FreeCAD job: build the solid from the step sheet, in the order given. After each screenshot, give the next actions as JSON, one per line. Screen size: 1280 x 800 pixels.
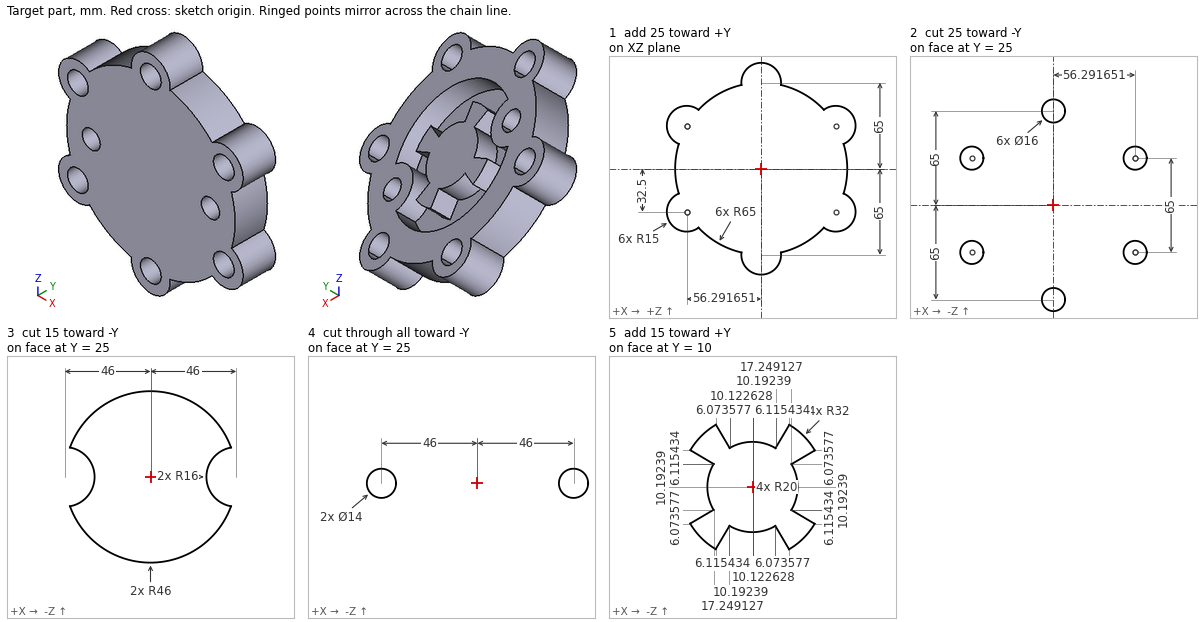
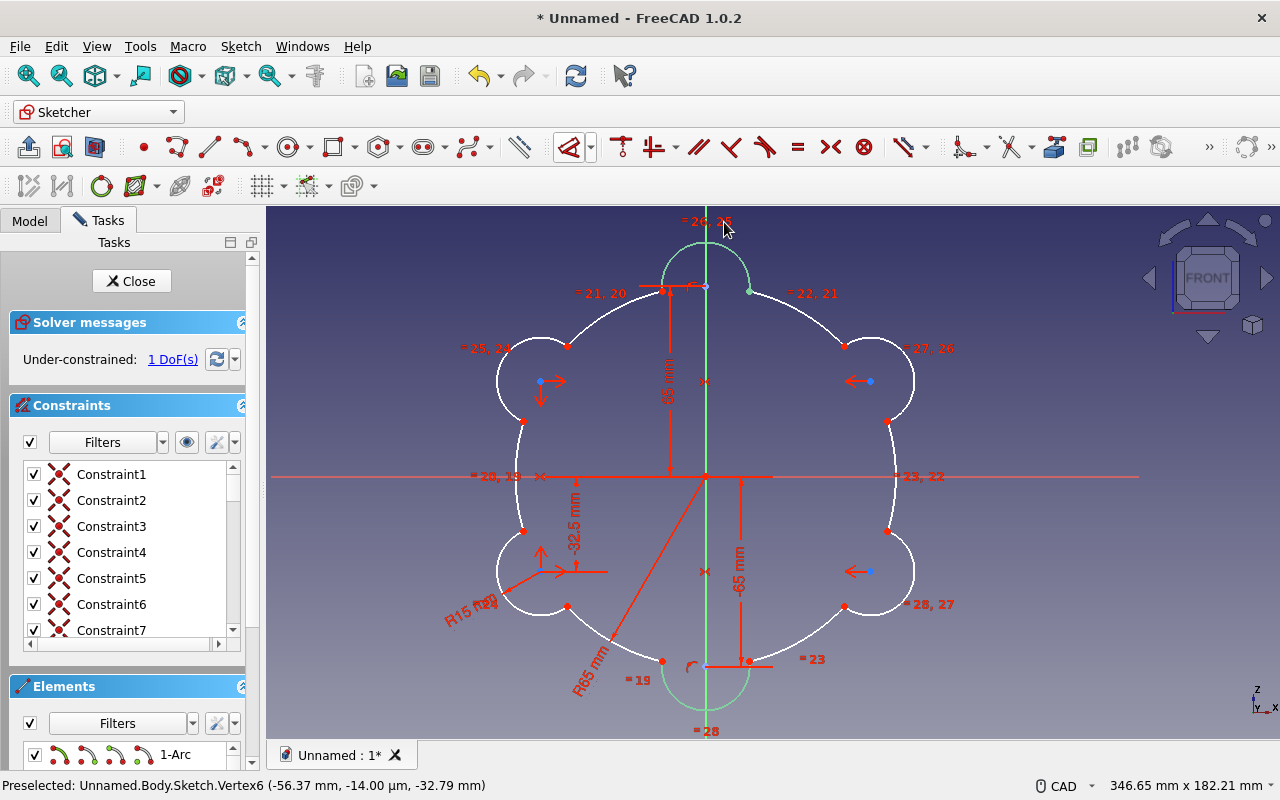
{"action": "left_click", "coordinate": [541, 572]}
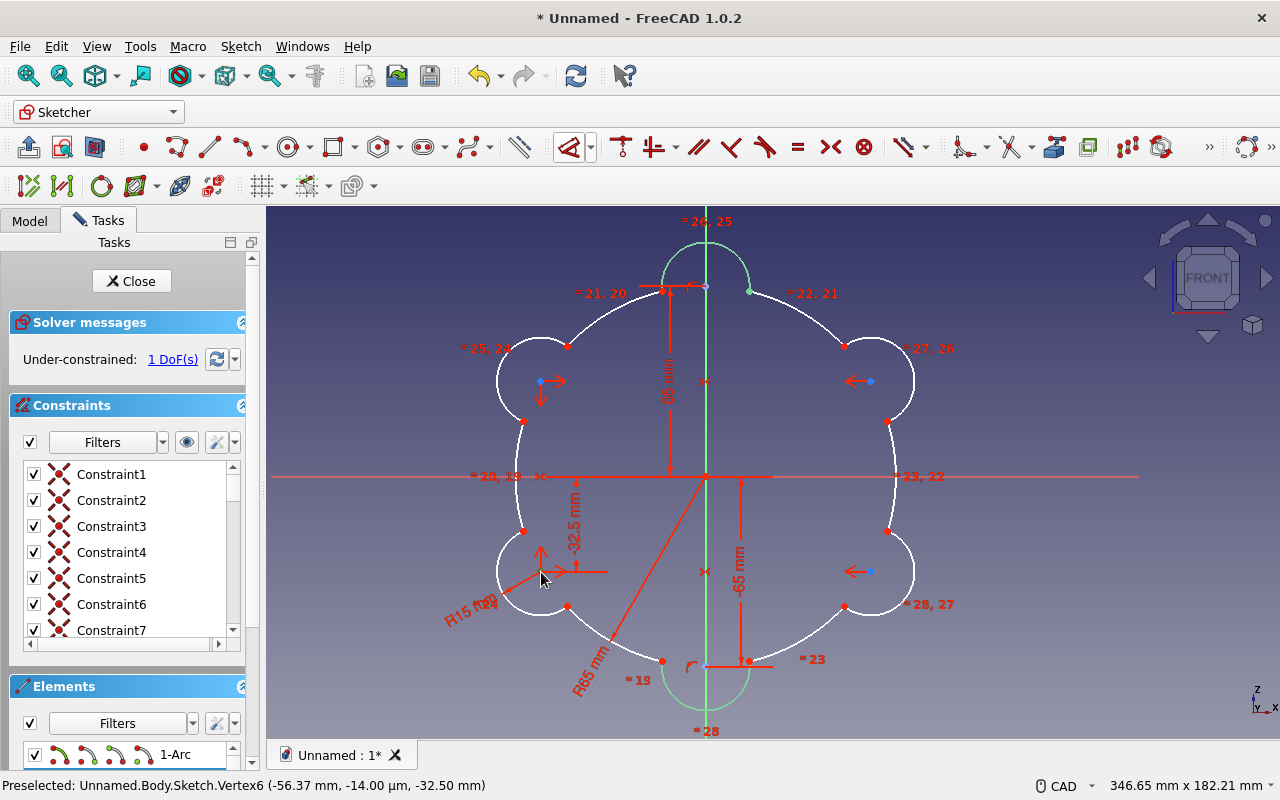
{"action": "left_click", "coordinate": [590, 148]}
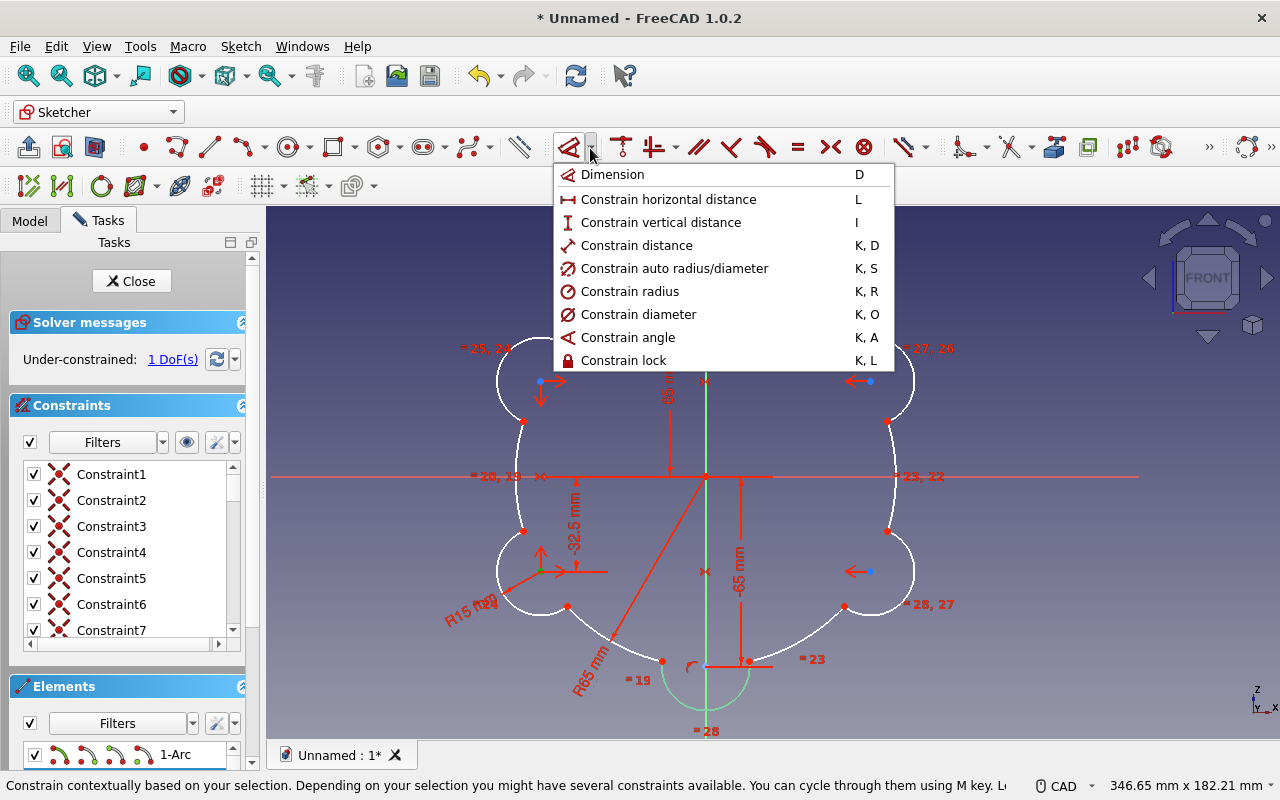
{"action": "left_click", "coordinate": [724, 200]}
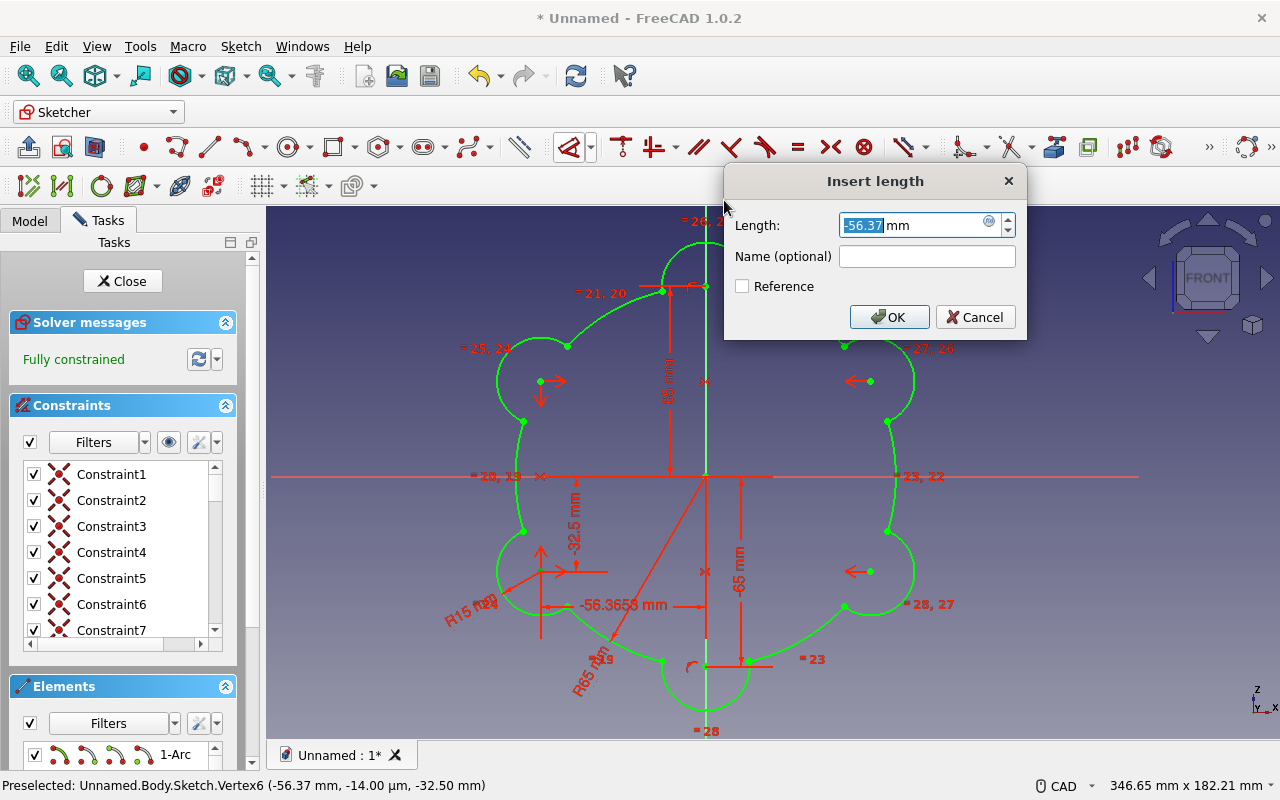
{"action": "type", "text": "-56.291651"}
{"action": "key", "text": "Return"}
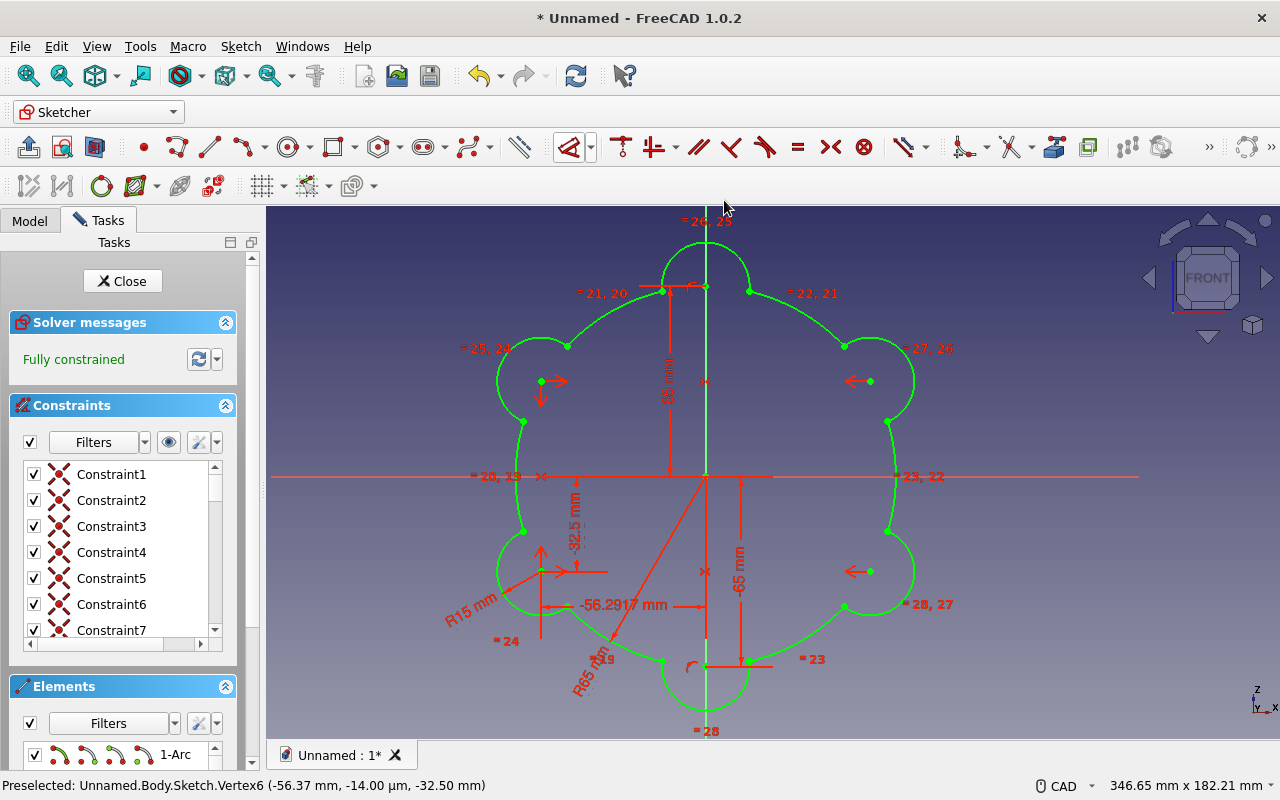
{"action": "left_click", "coordinate": [123, 281]}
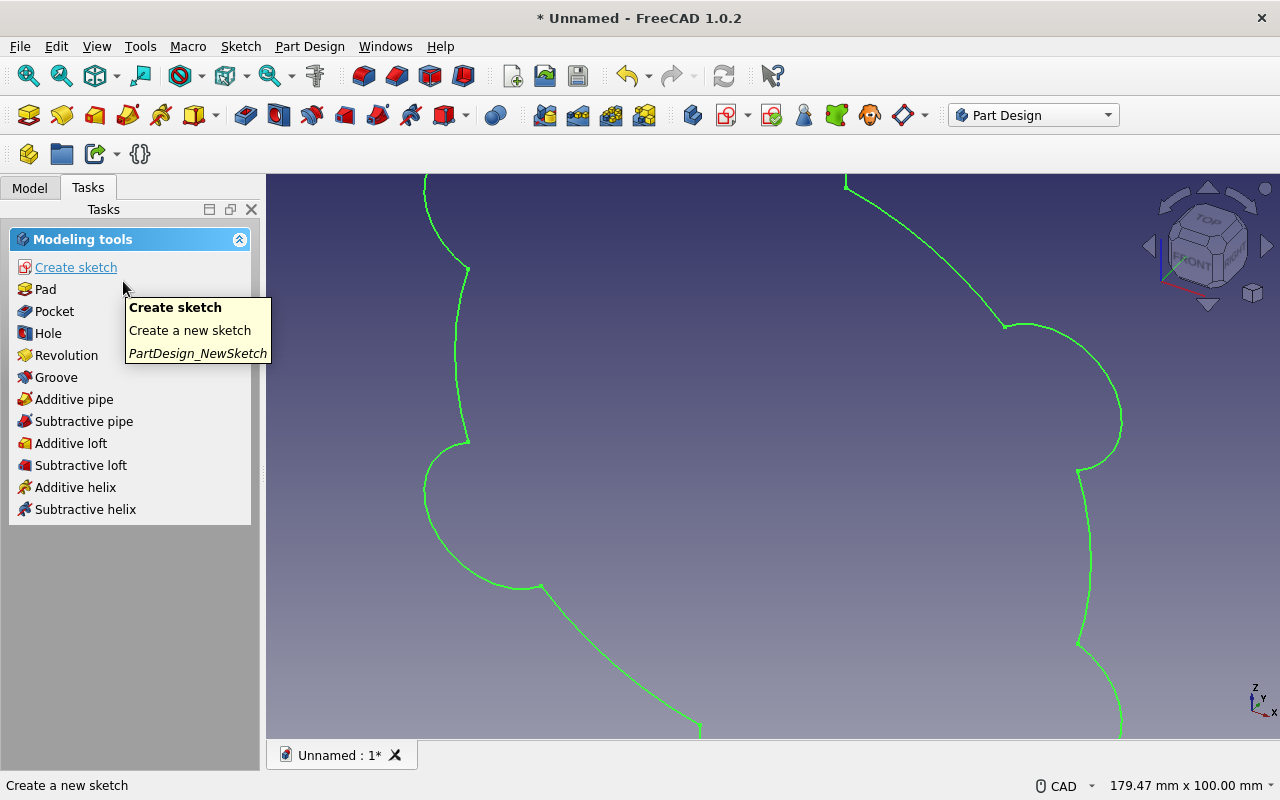
{"action": "left_click", "coordinate": [29, 116]}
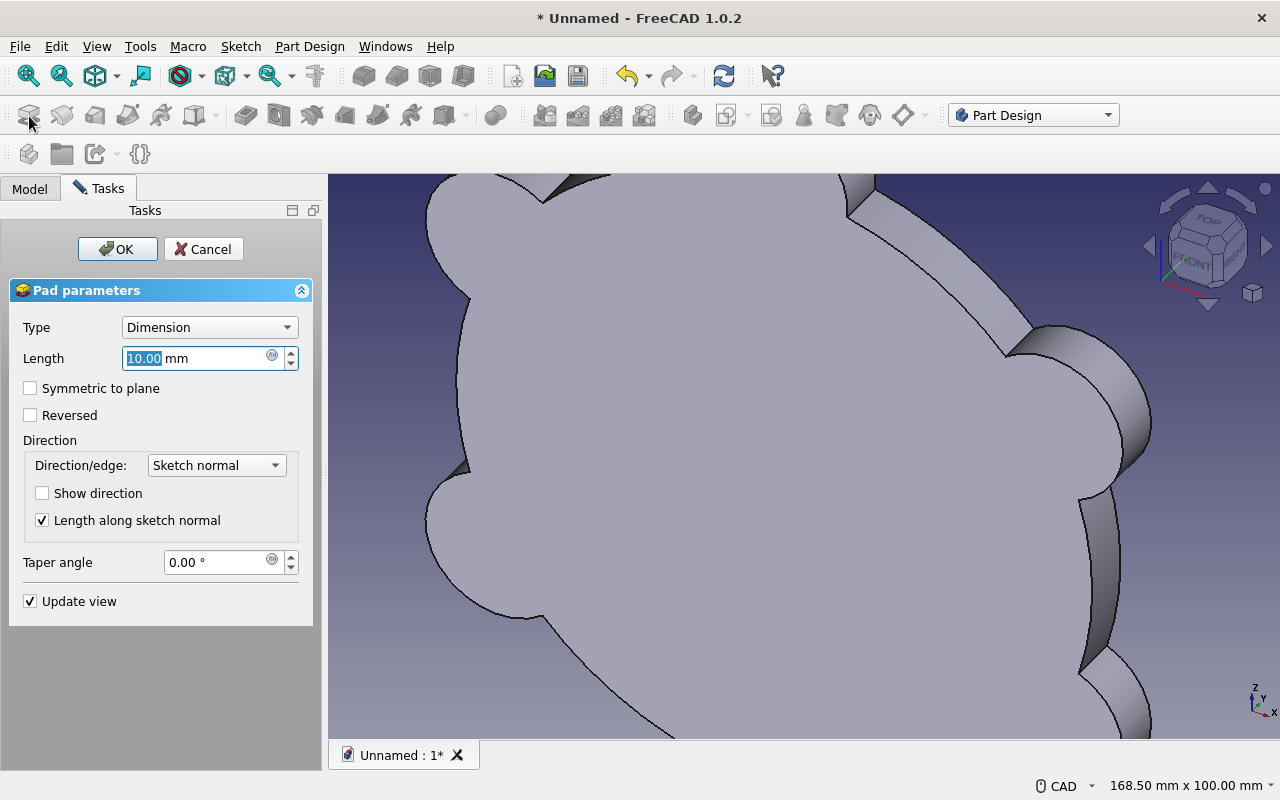
{"action": "type", "text": "25"}
{"action": "key", "text": "Tab"}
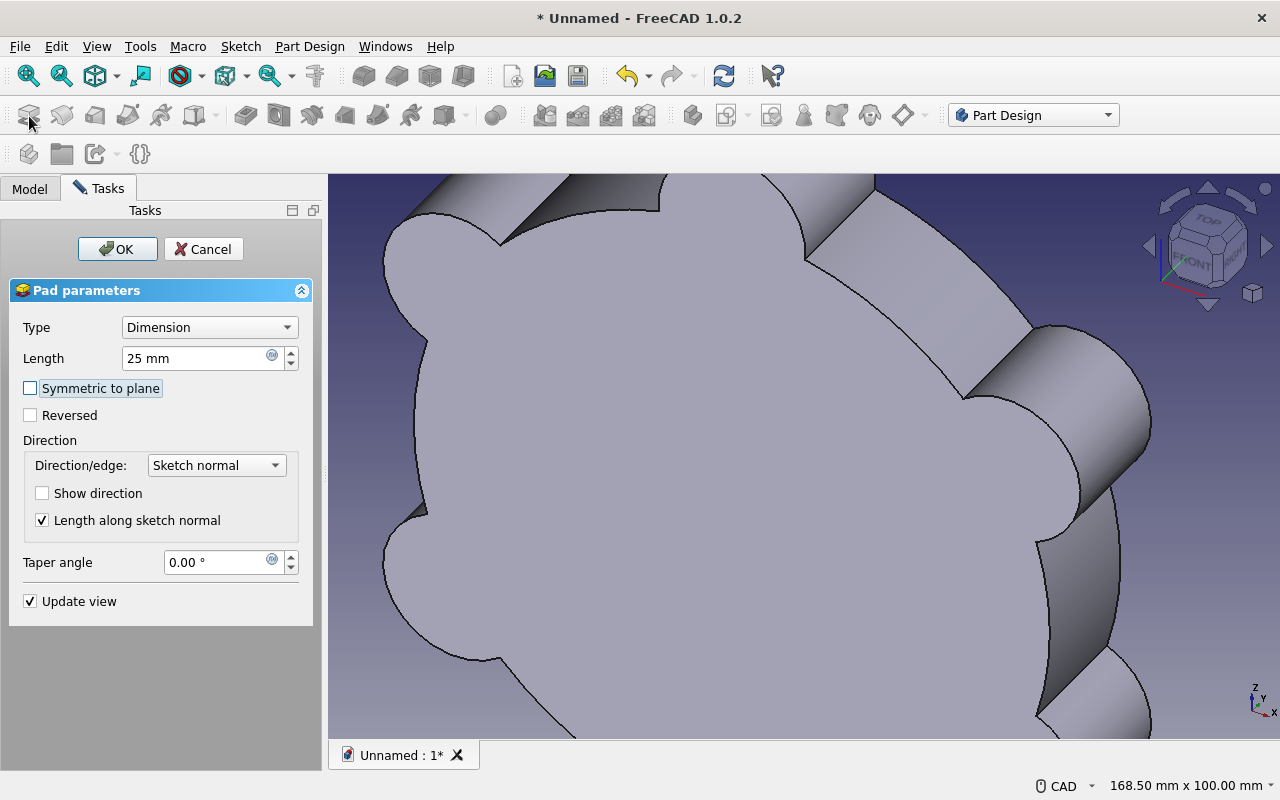
{"action": "left_click", "coordinate": [31, 415]}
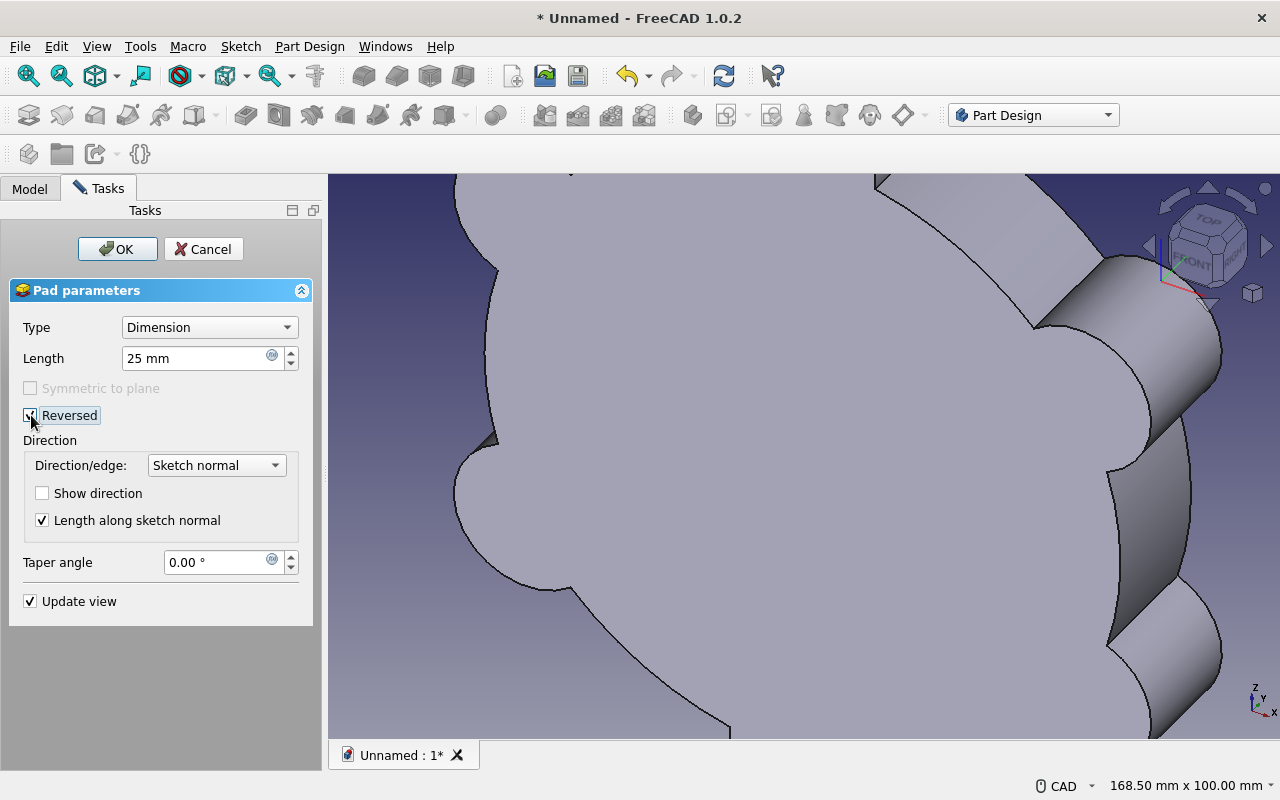
{"action": "left_click", "coordinate": [118, 249]}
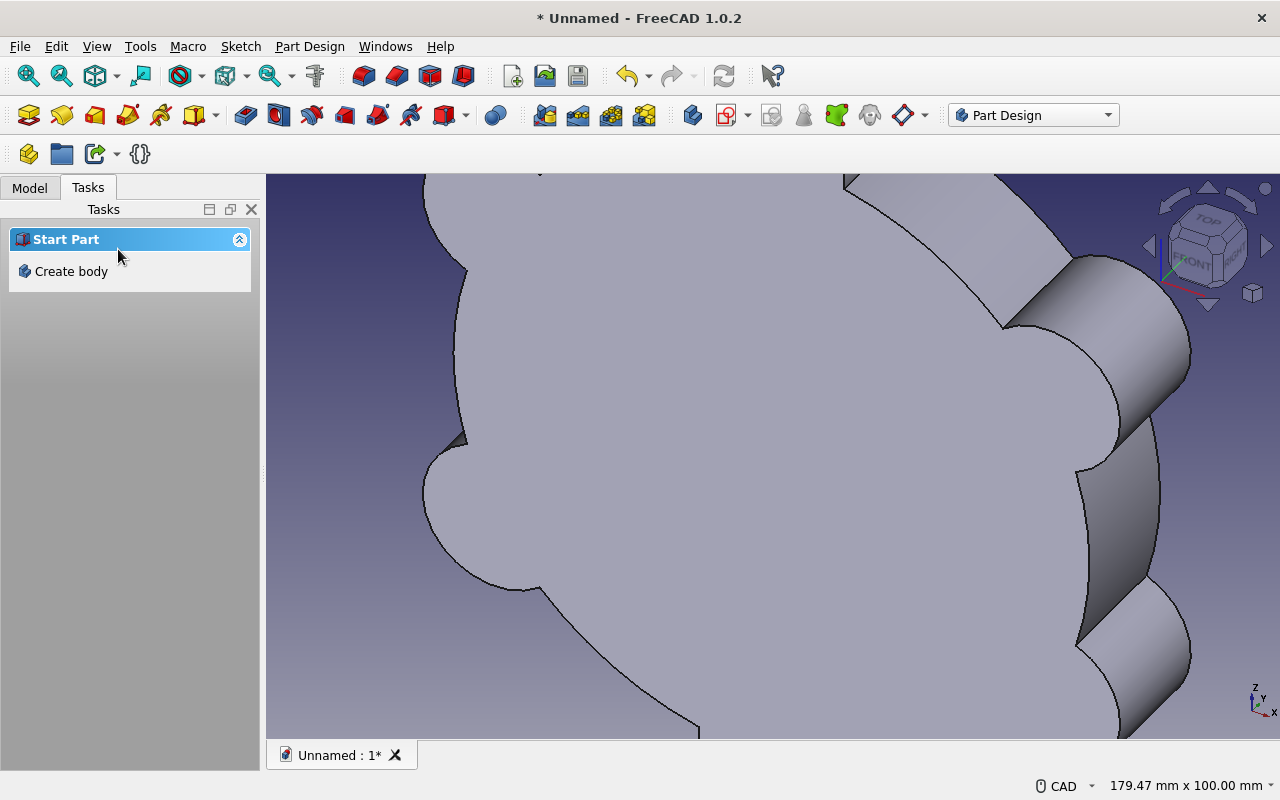
{"action": "left_click", "coordinate": [29, 76]}